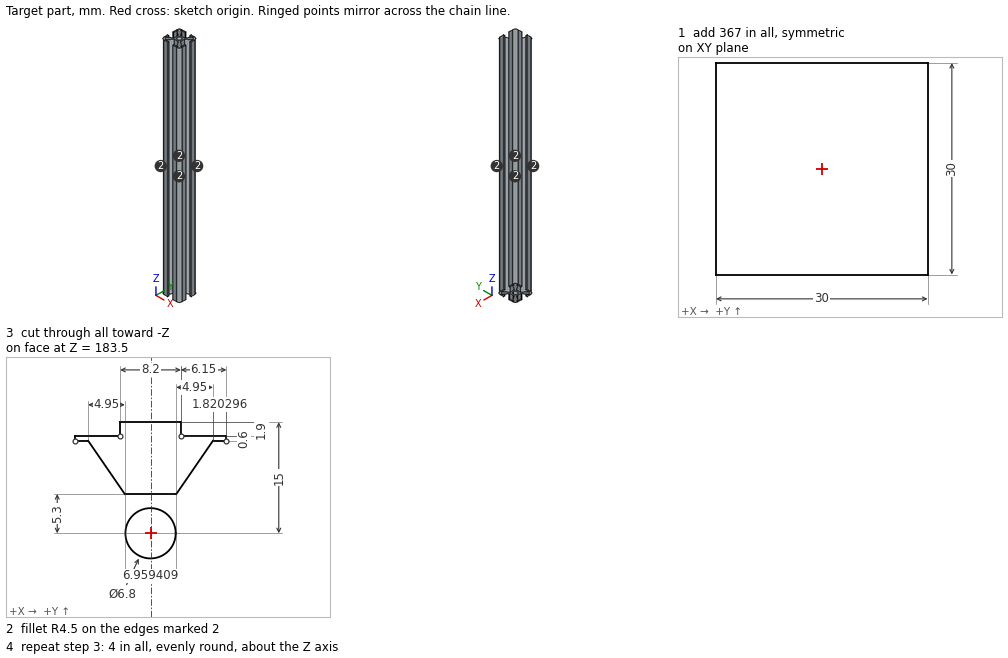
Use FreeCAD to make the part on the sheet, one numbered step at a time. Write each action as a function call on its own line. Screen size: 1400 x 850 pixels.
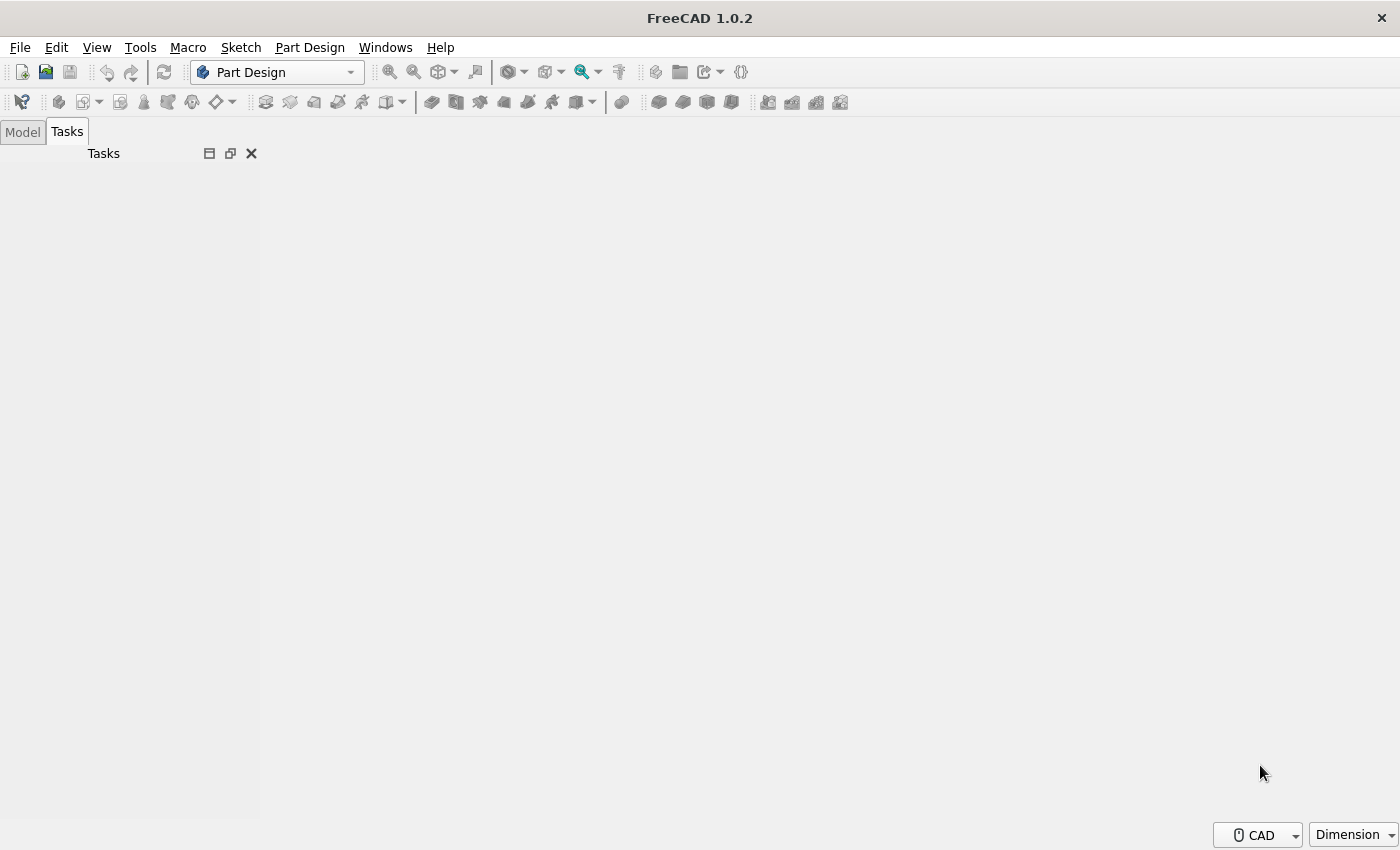
key(ctrl+n)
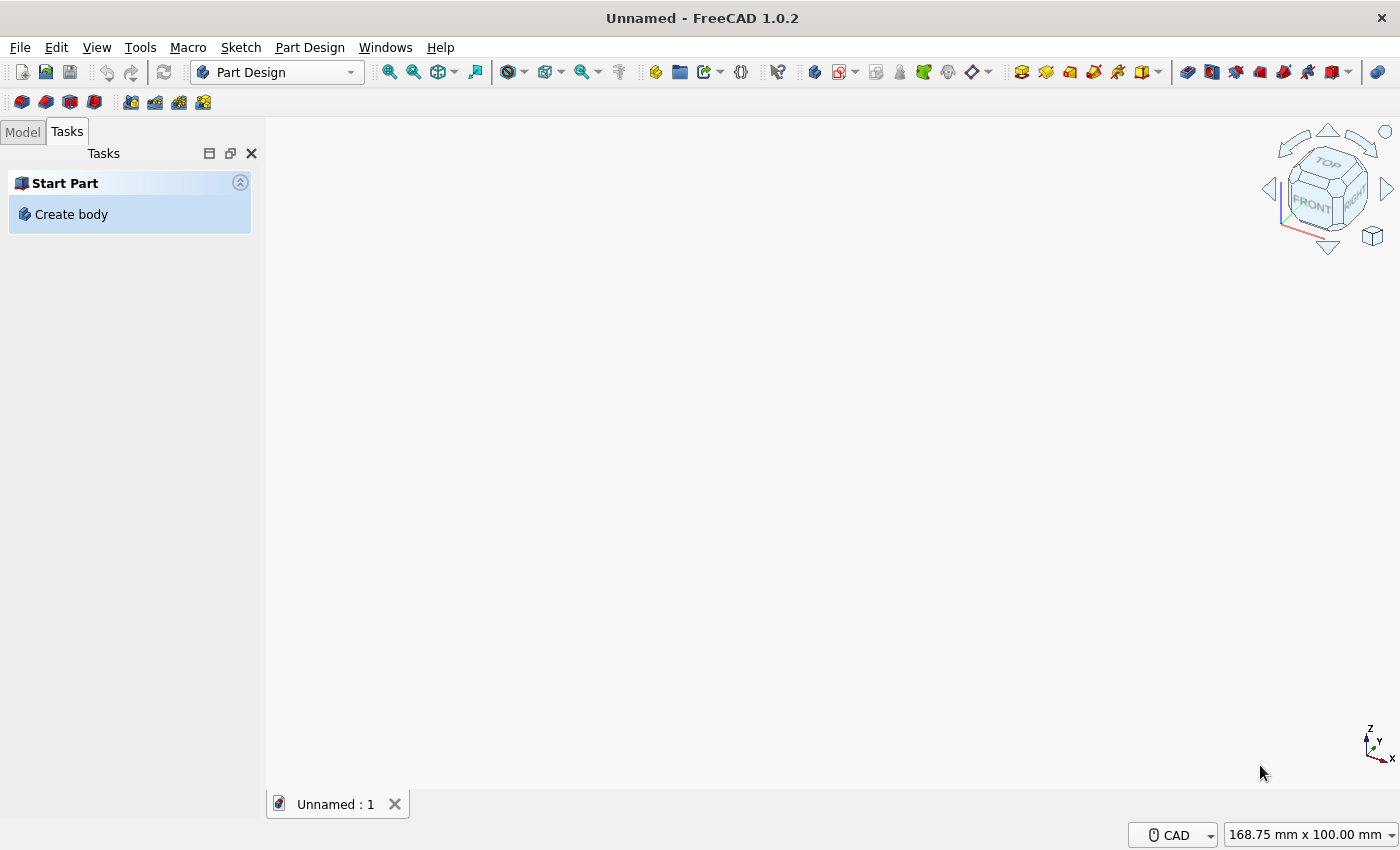
click(840, 72)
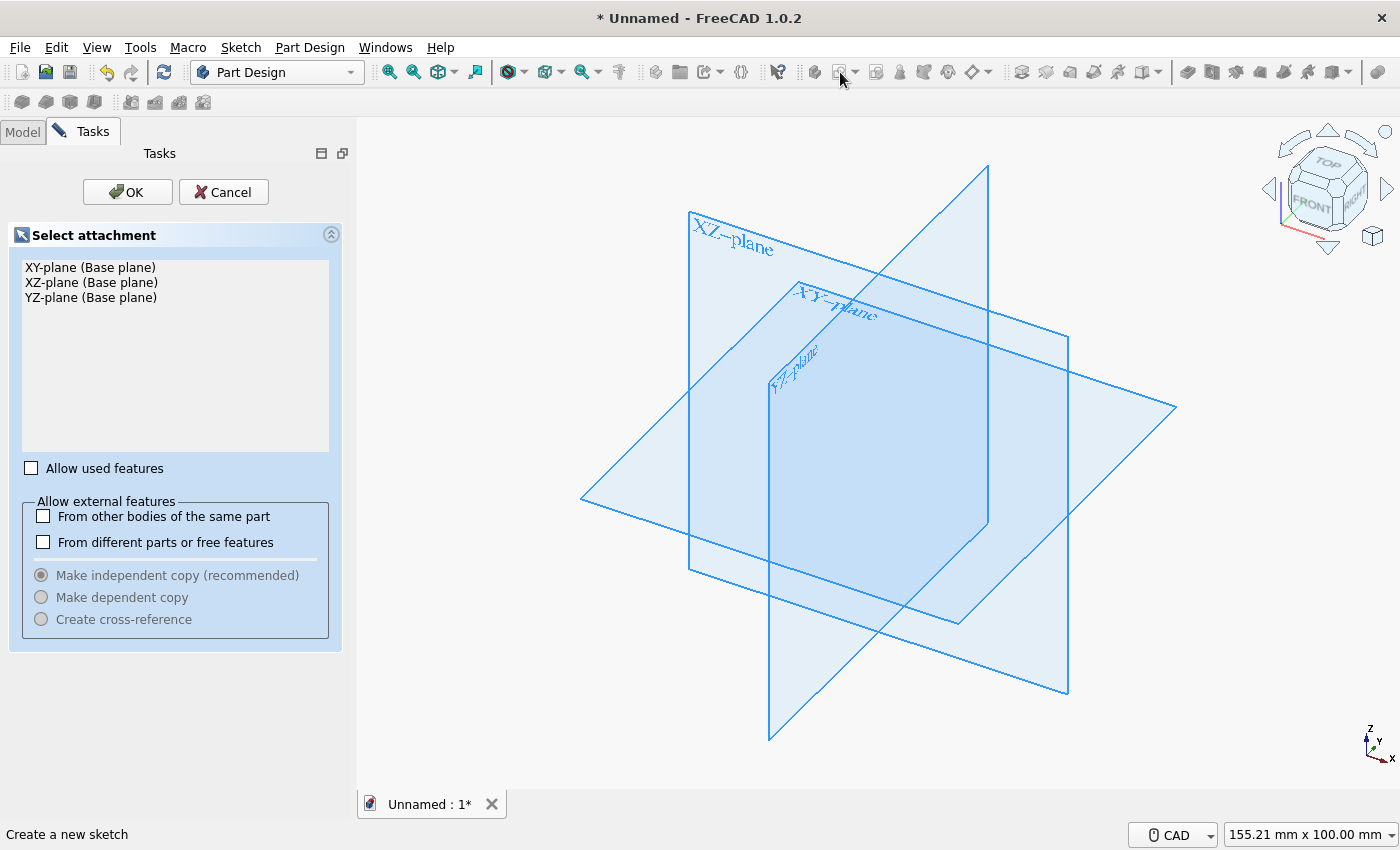
click(82, 268)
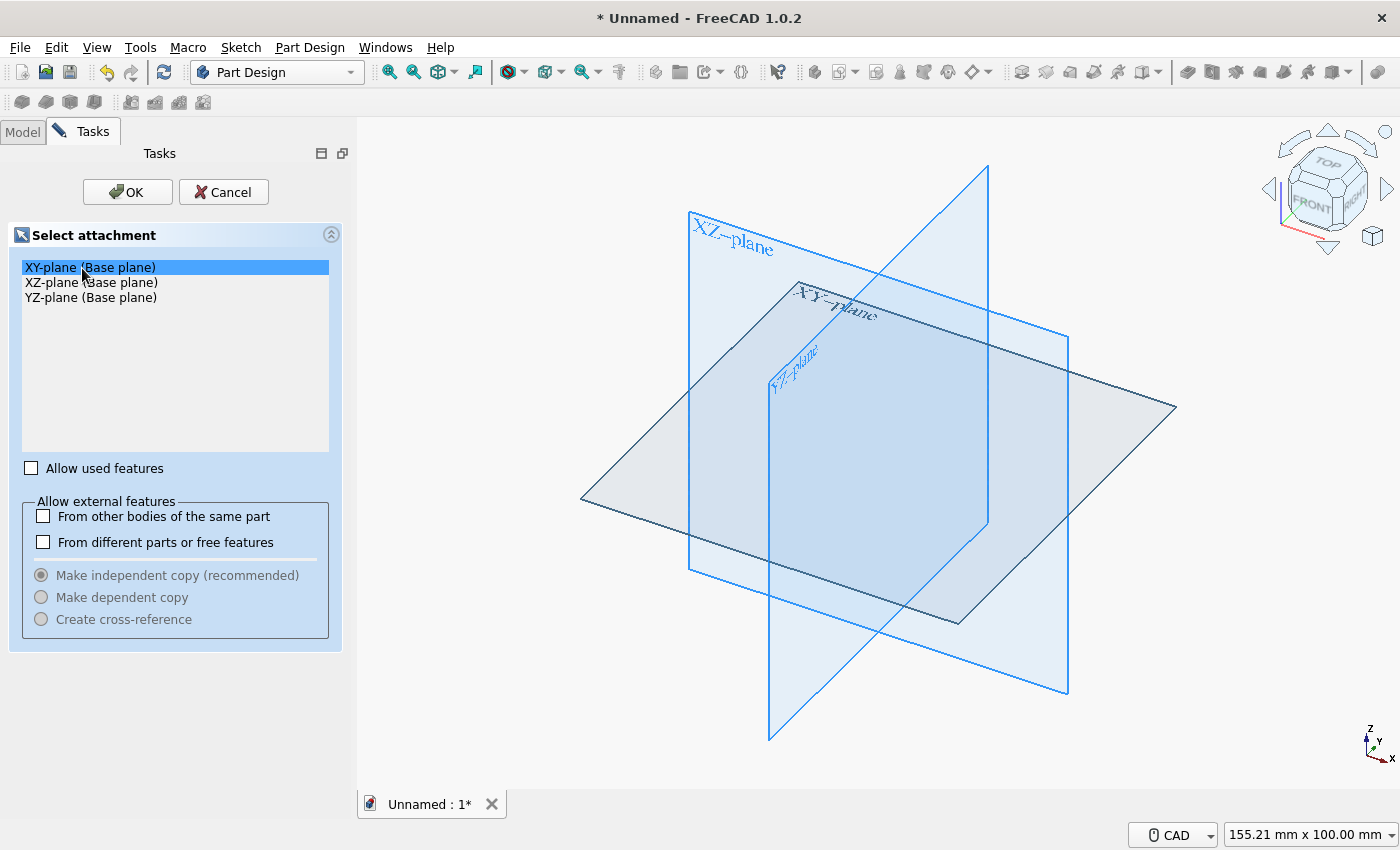
click(128, 192)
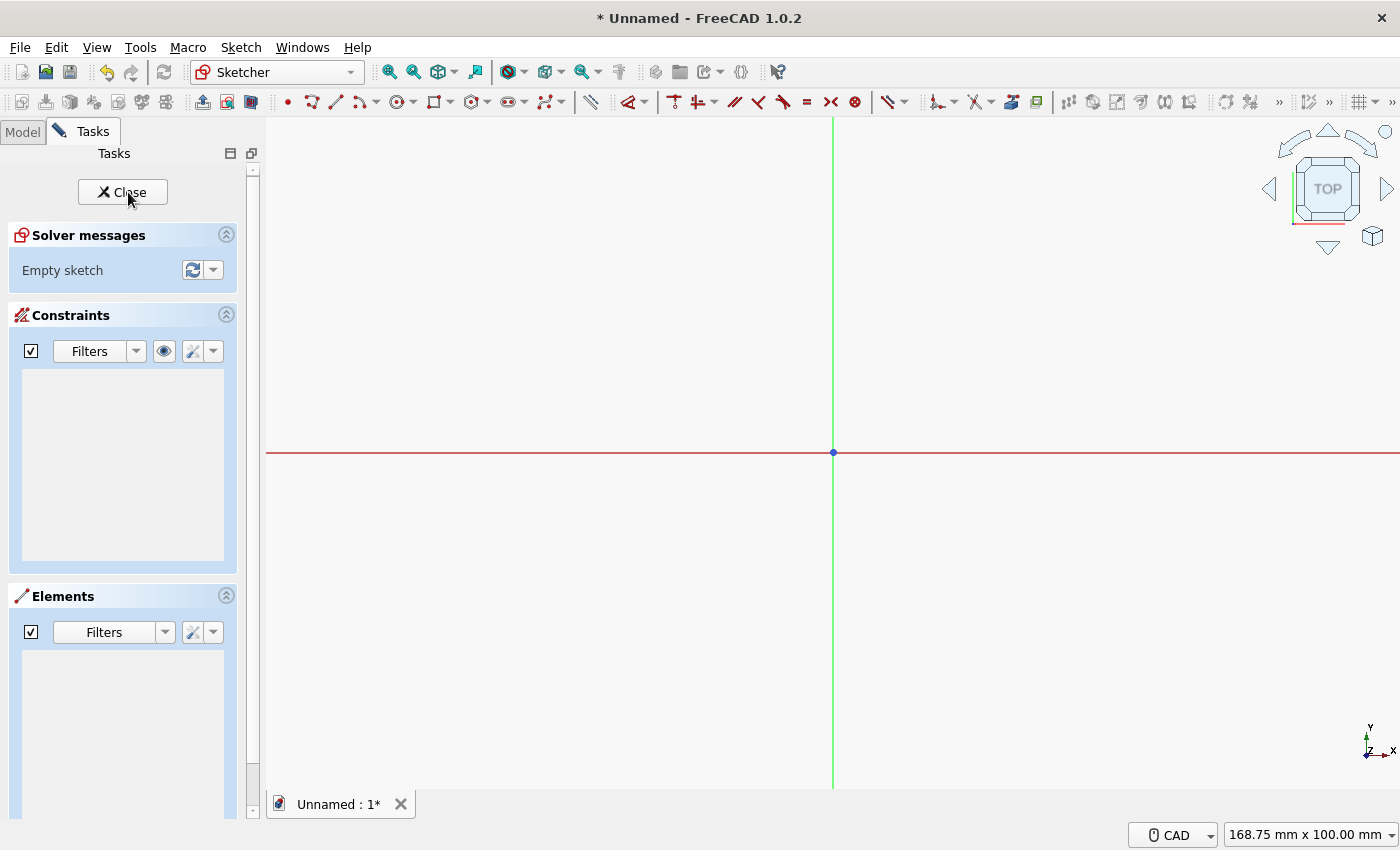
scroll(889, 453, up, 4)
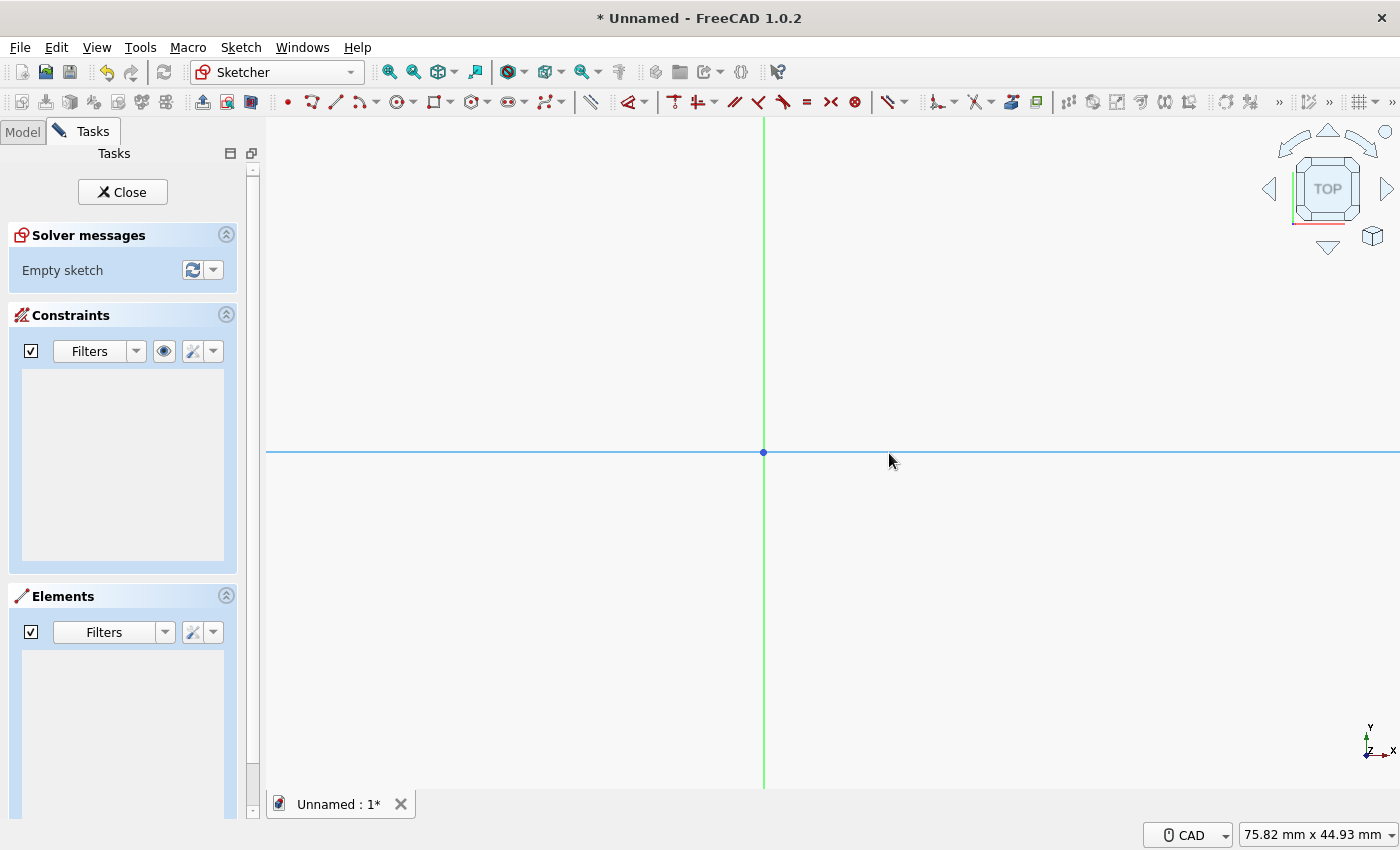
key(g)
key(v)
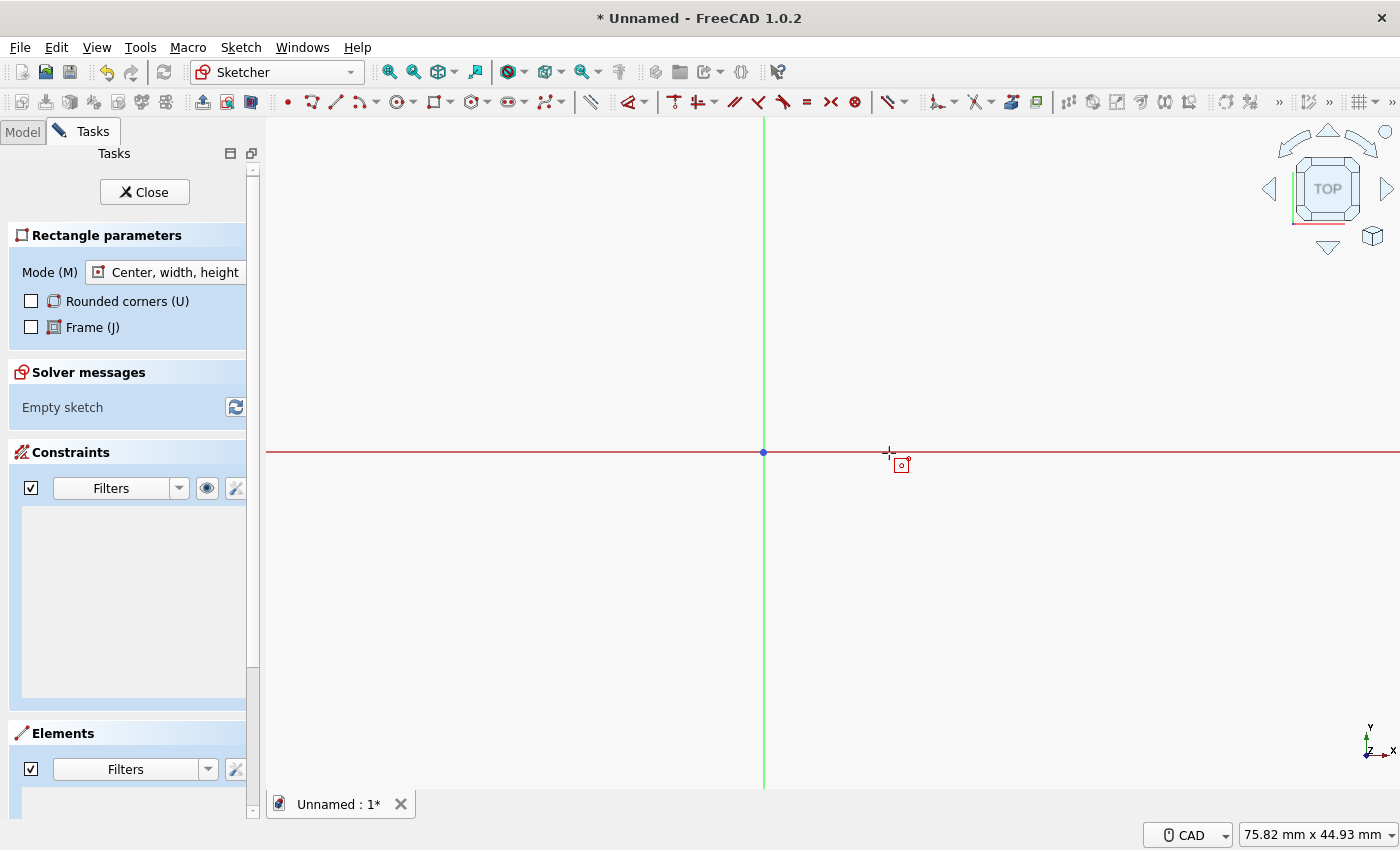
click(764, 452)
click(988, 228)
key(Escape)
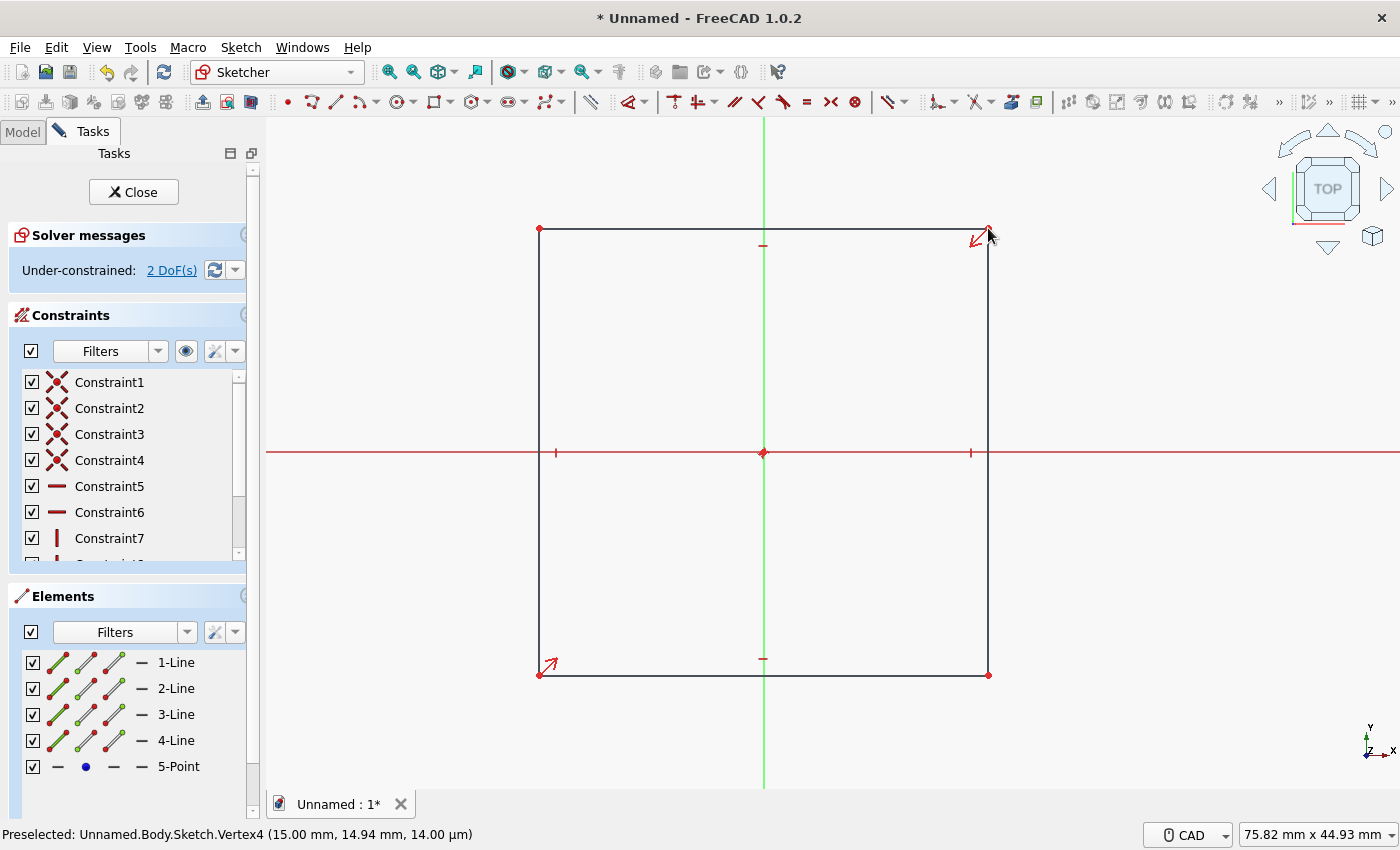
key(d)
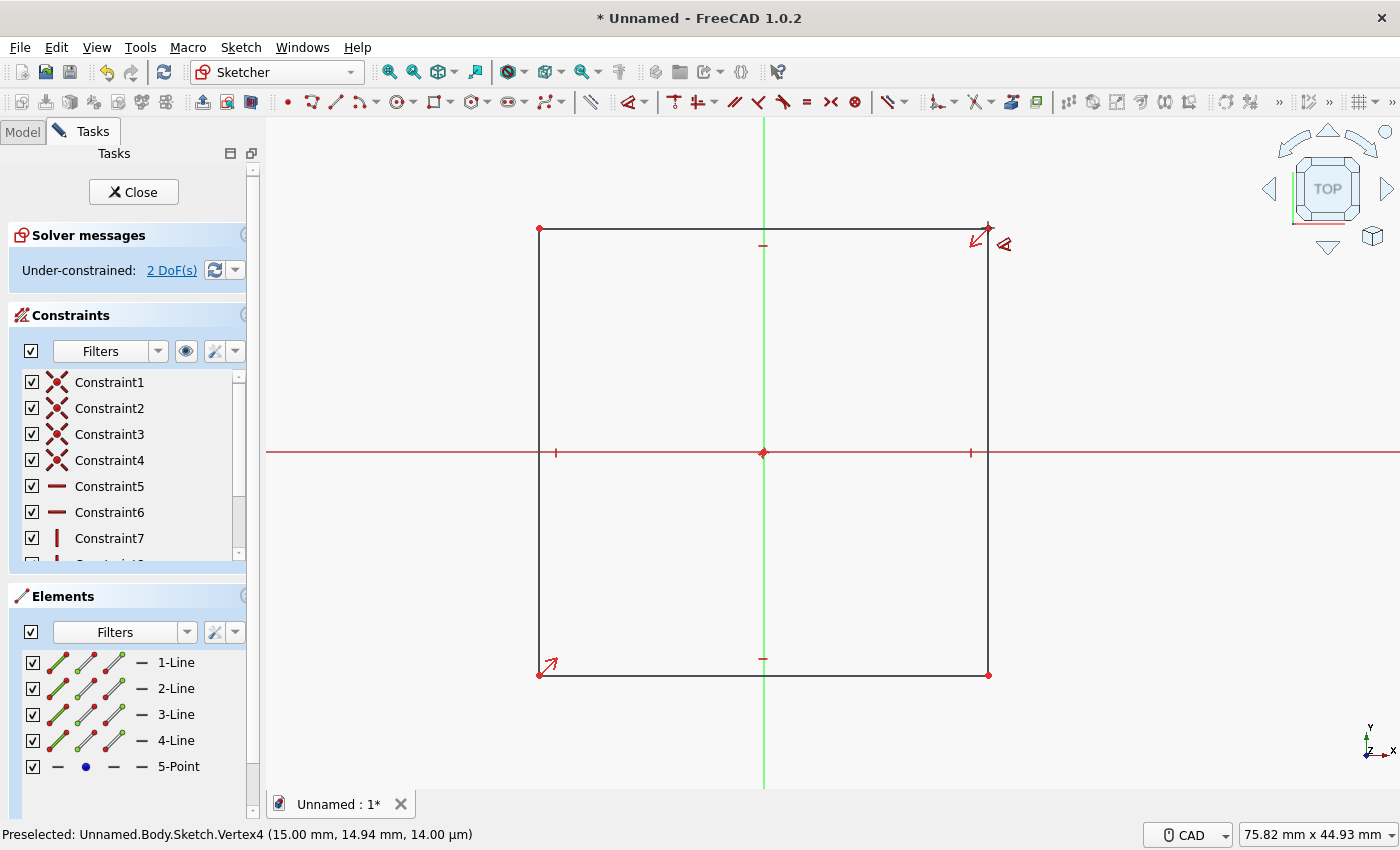
click(674, 676)
click(661, 710)